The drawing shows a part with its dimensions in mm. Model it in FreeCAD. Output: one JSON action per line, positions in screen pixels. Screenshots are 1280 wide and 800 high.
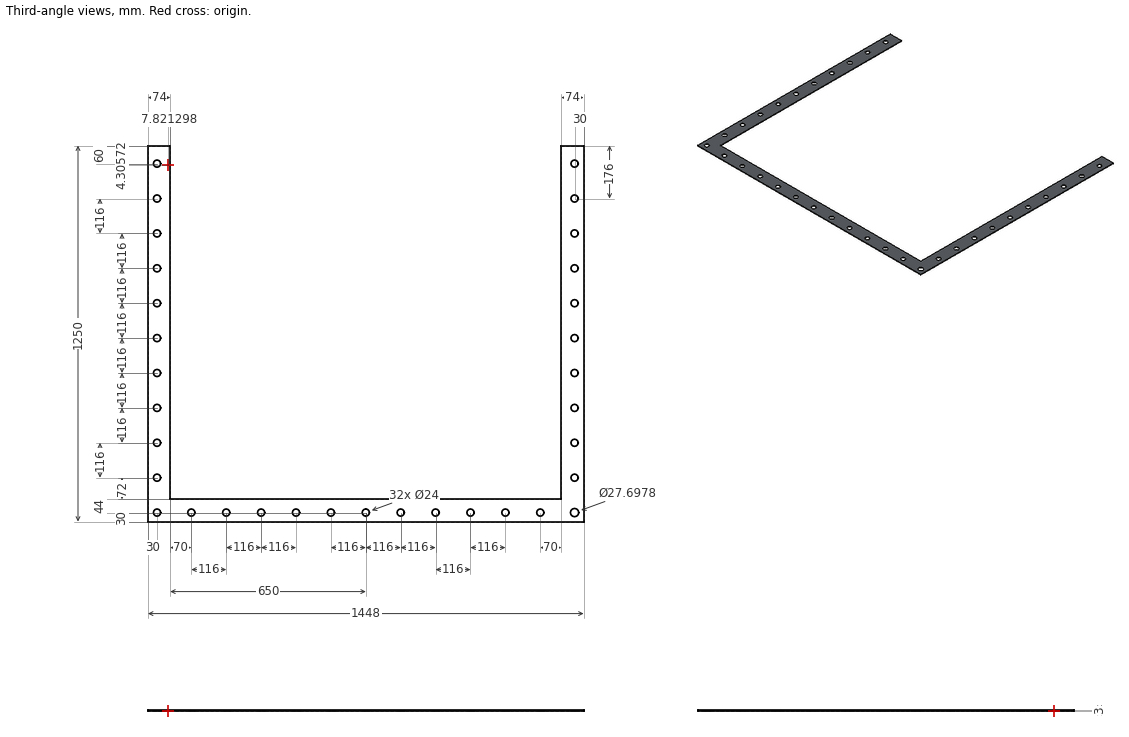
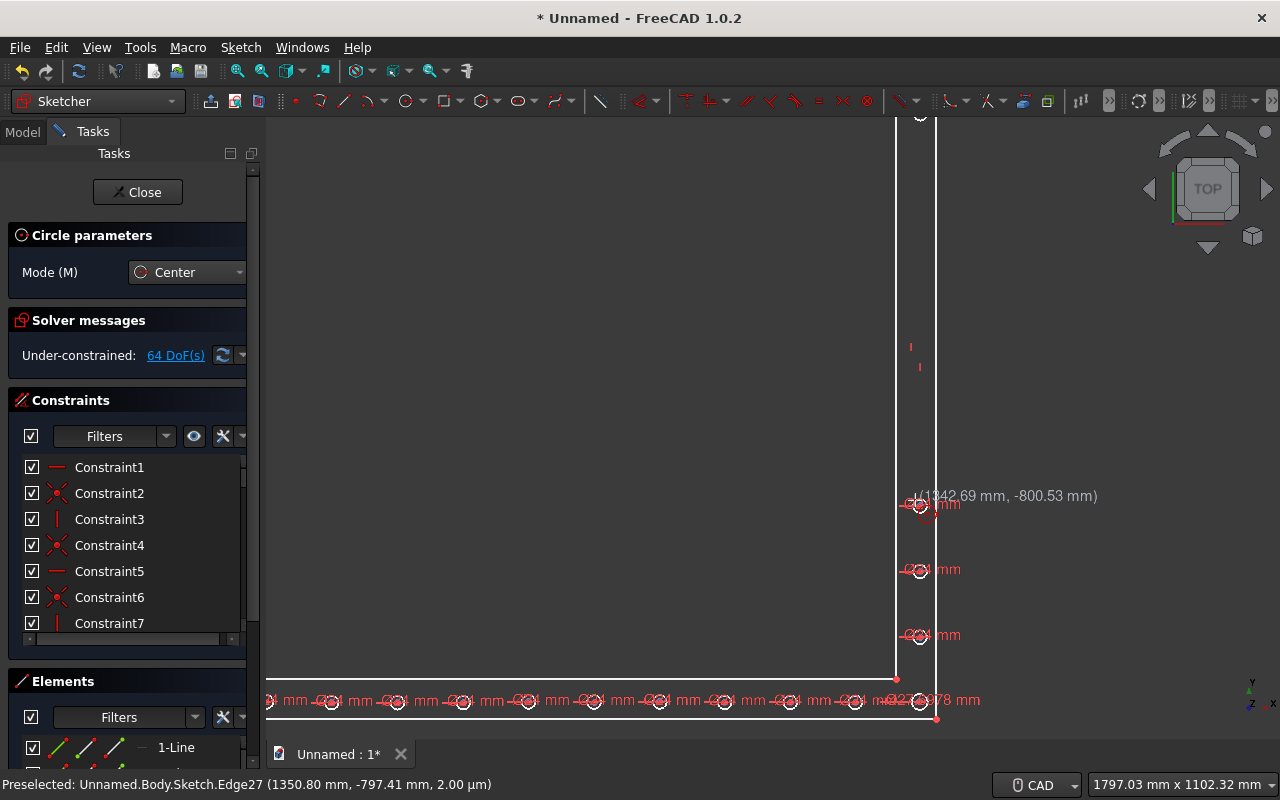
{"action": "scroll", "coordinate": [920, 440], "scroll_direction": "up", "scroll_amount": 7}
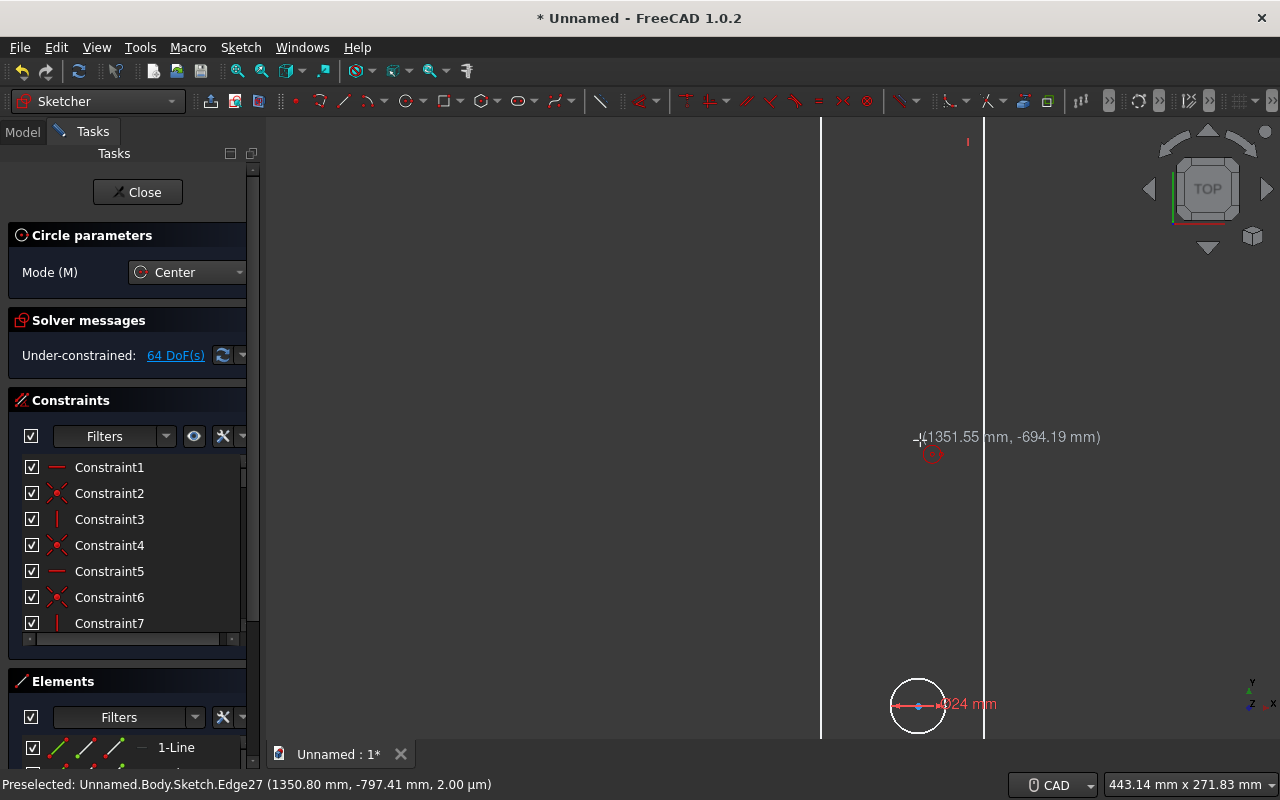
{"action": "scroll", "coordinate": [920, 474], "scroll_direction": "down", "scroll_amount": 10}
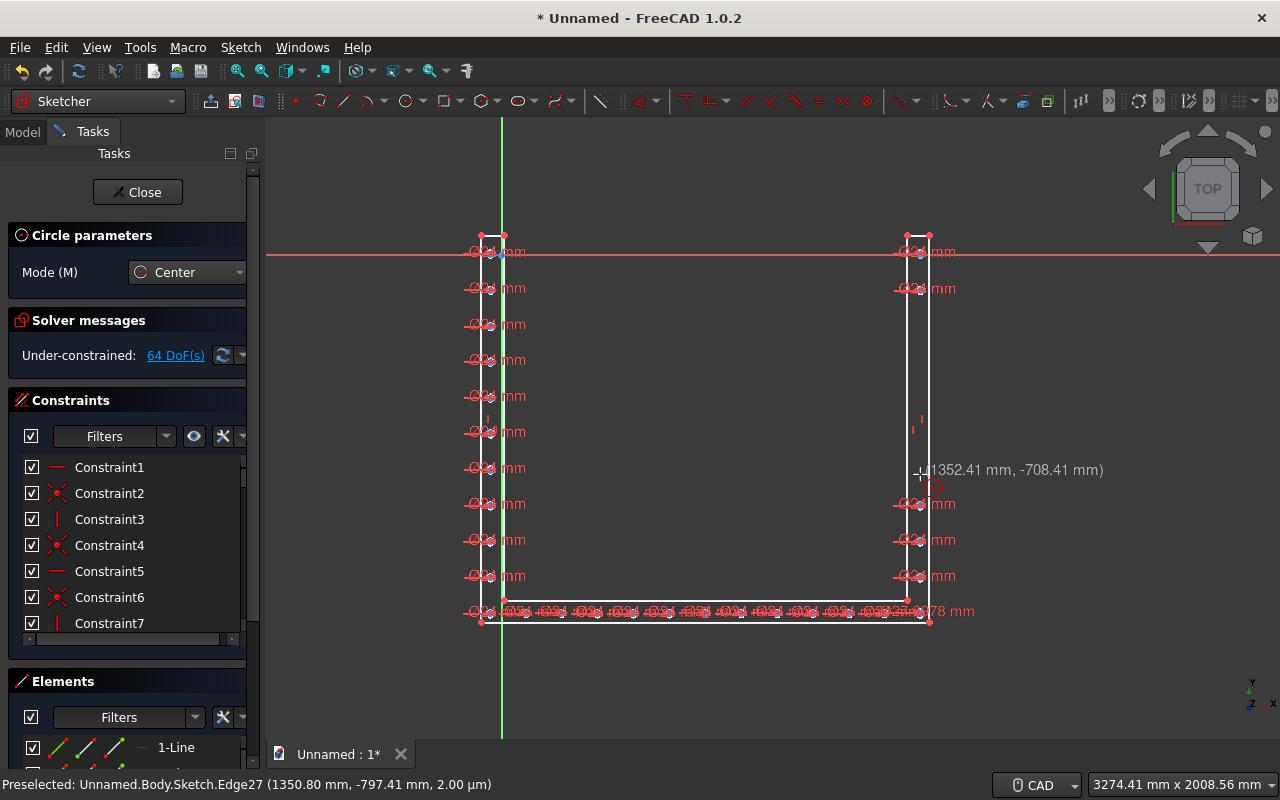
{"action": "scroll", "coordinate": [920, 469], "scroll_direction": "up", "scroll_amount": 3}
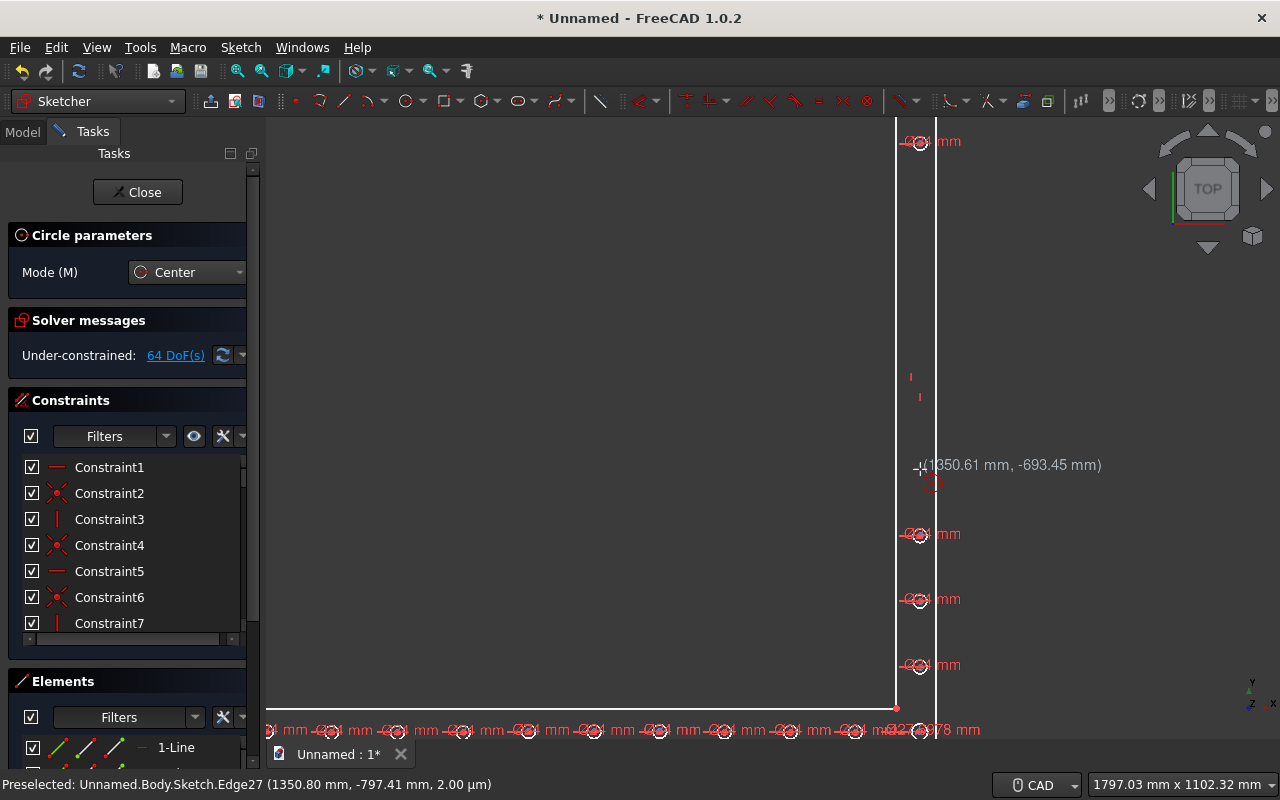
{"action": "left_click", "coordinate": [920, 469]}
{"action": "mouse_move", "coordinate": [915, 465]}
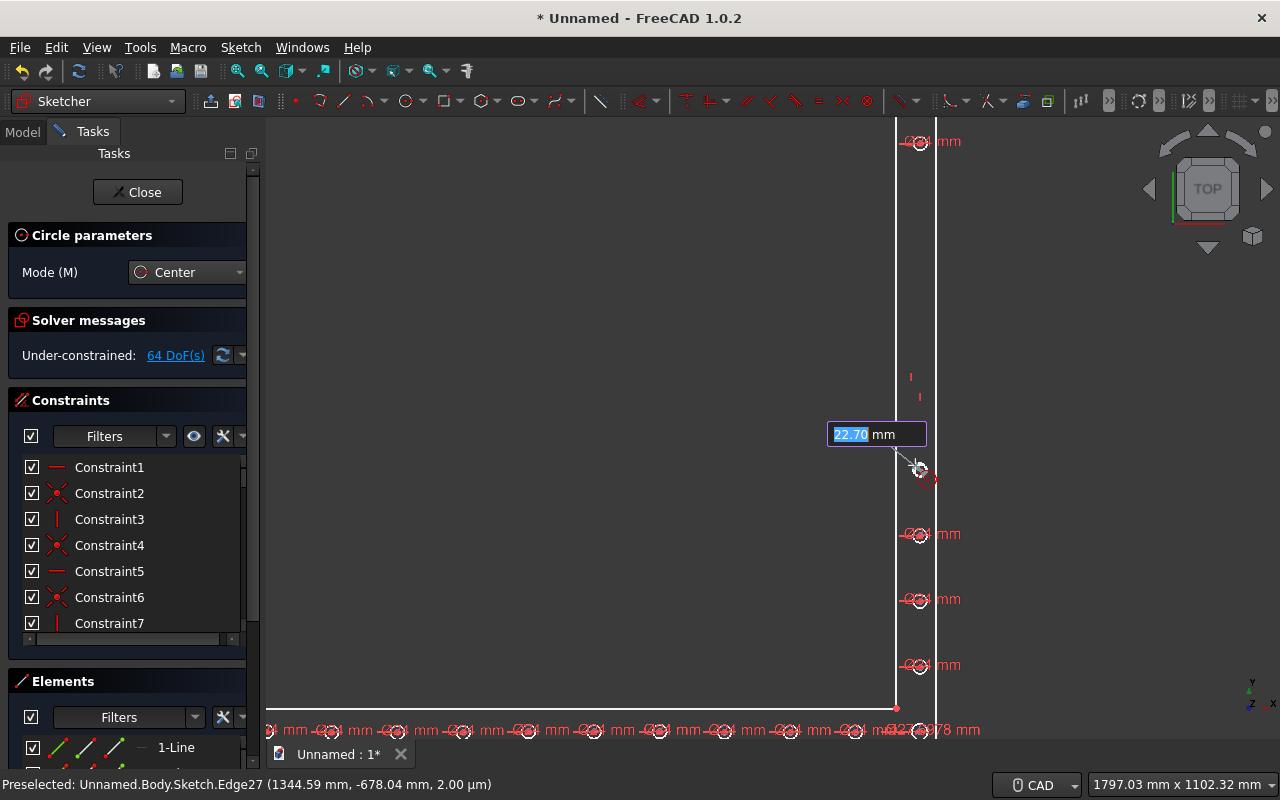
{"action": "type", "text": "24"}
{"action": "key", "text": "Return"}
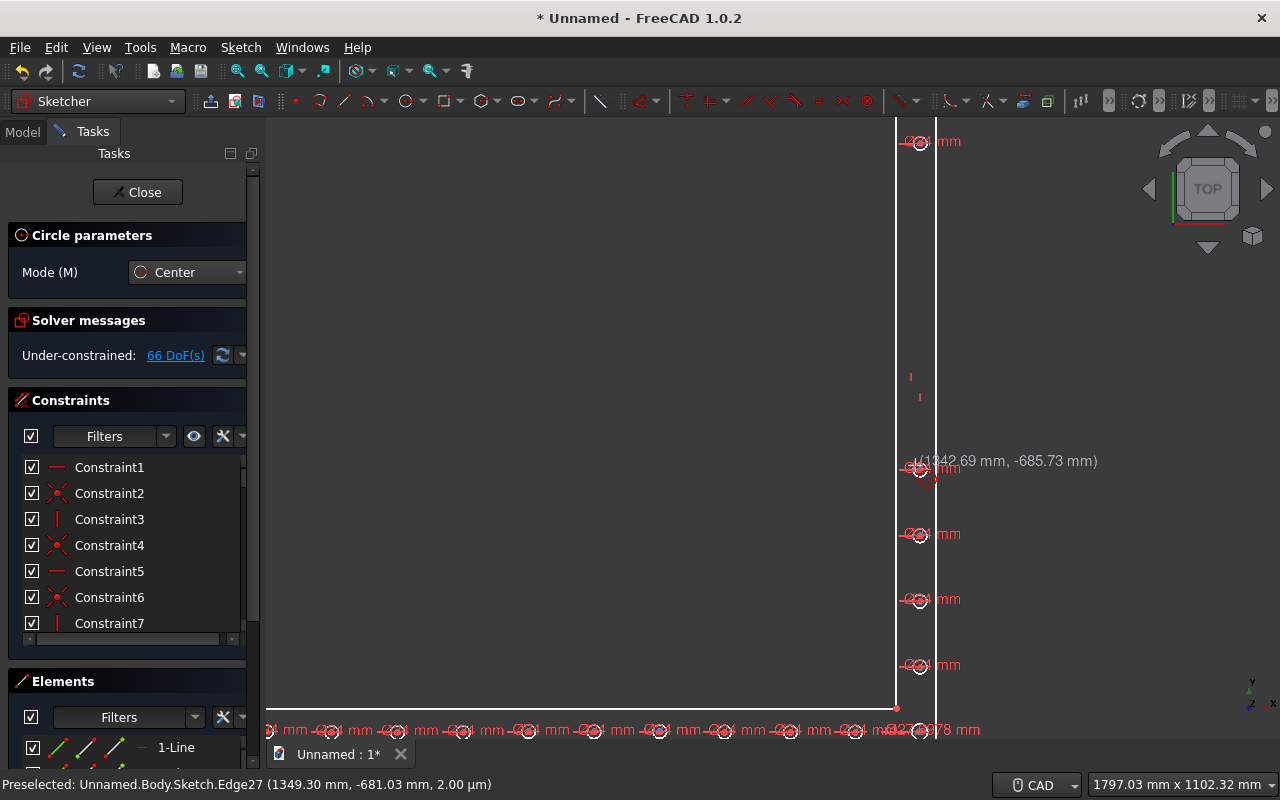
{"action": "scroll", "coordinate": [920, 404], "scroll_direction": "up", "scroll_amount": 7}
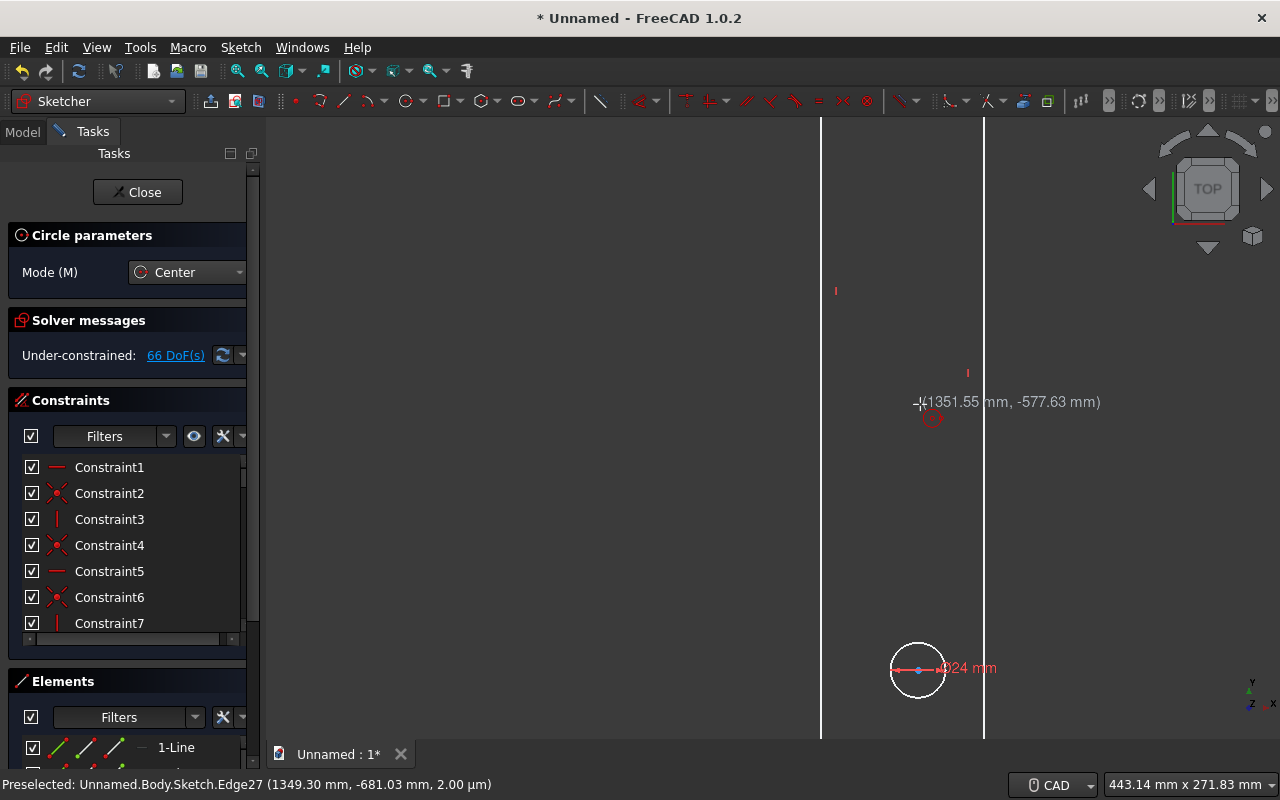
{"action": "scroll", "coordinate": [920, 437], "scroll_direction": "down", "scroll_amount": 10}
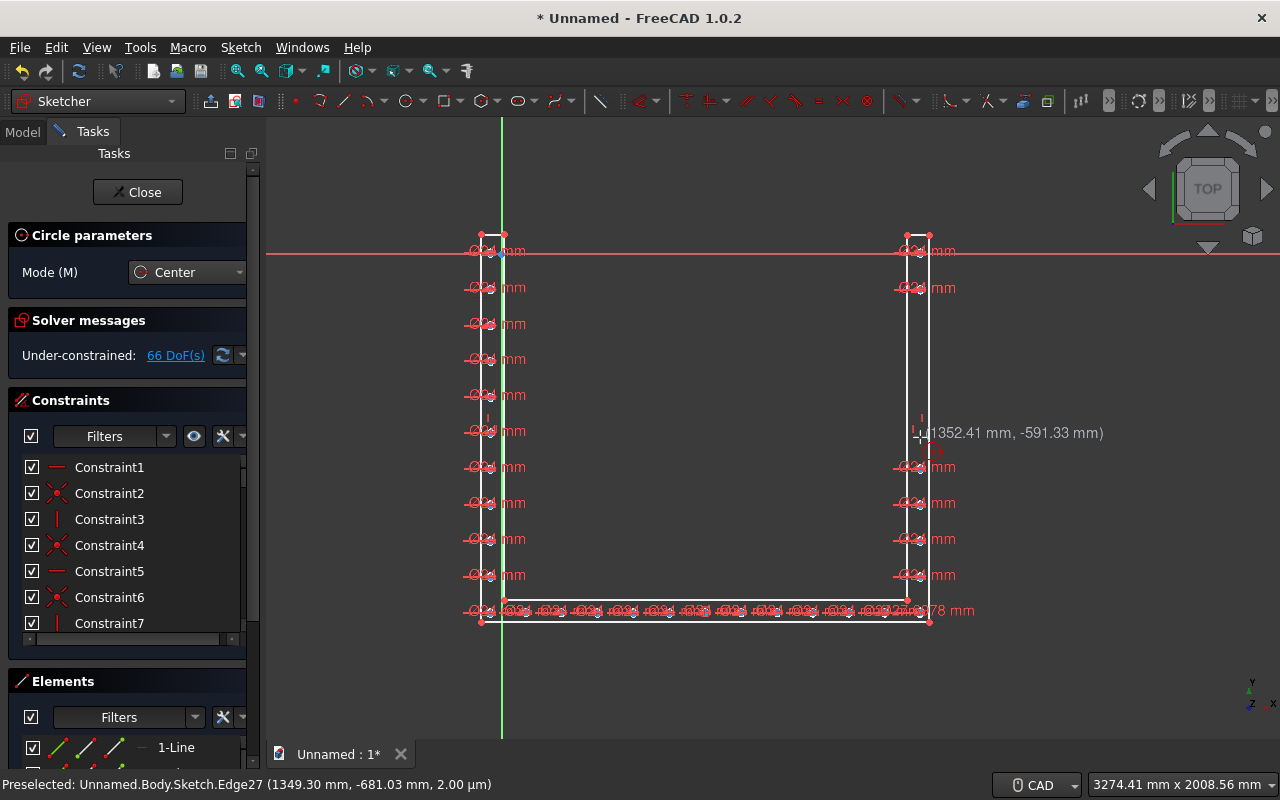
{"action": "scroll", "coordinate": [920, 433], "scroll_direction": "up", "scroll_amount": 3}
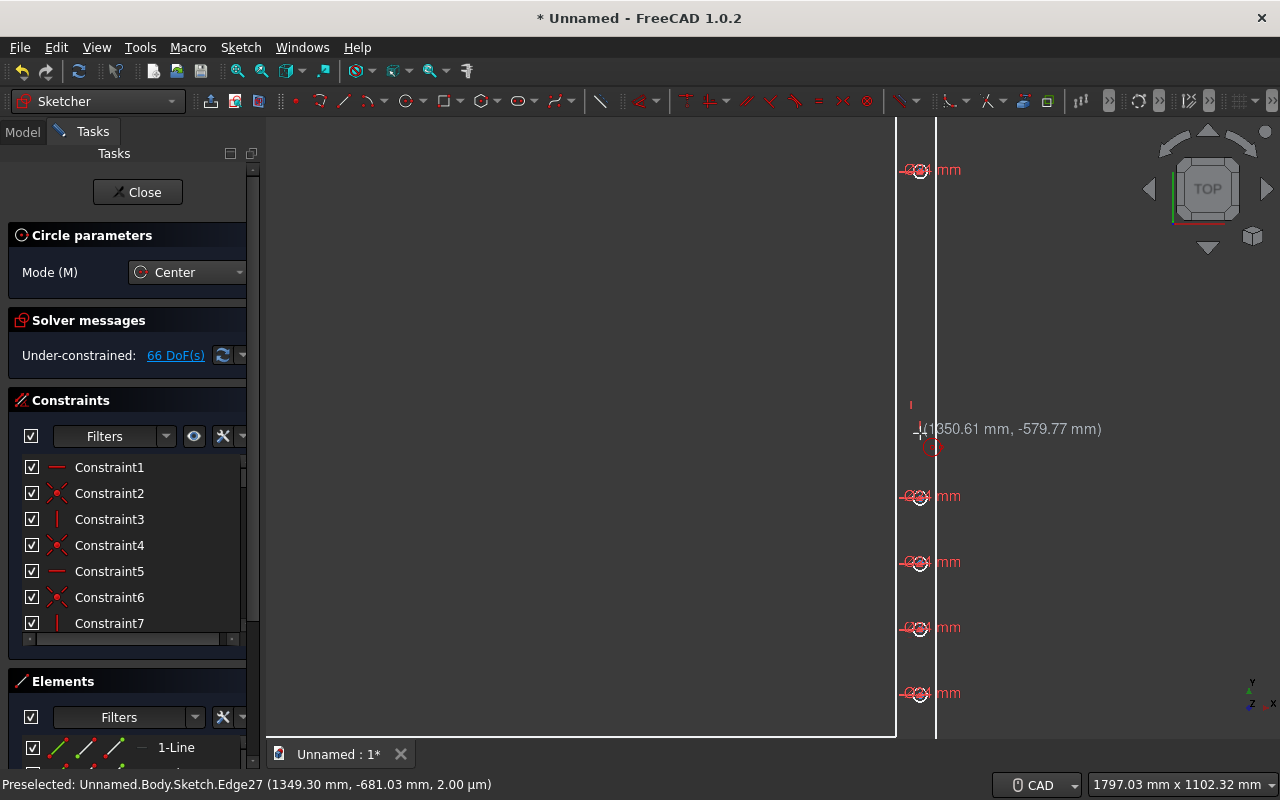
{"action": "left_click", "coordinate": [920, 432]}
{"action": "mouse_move", "coordinate": [915, 427]}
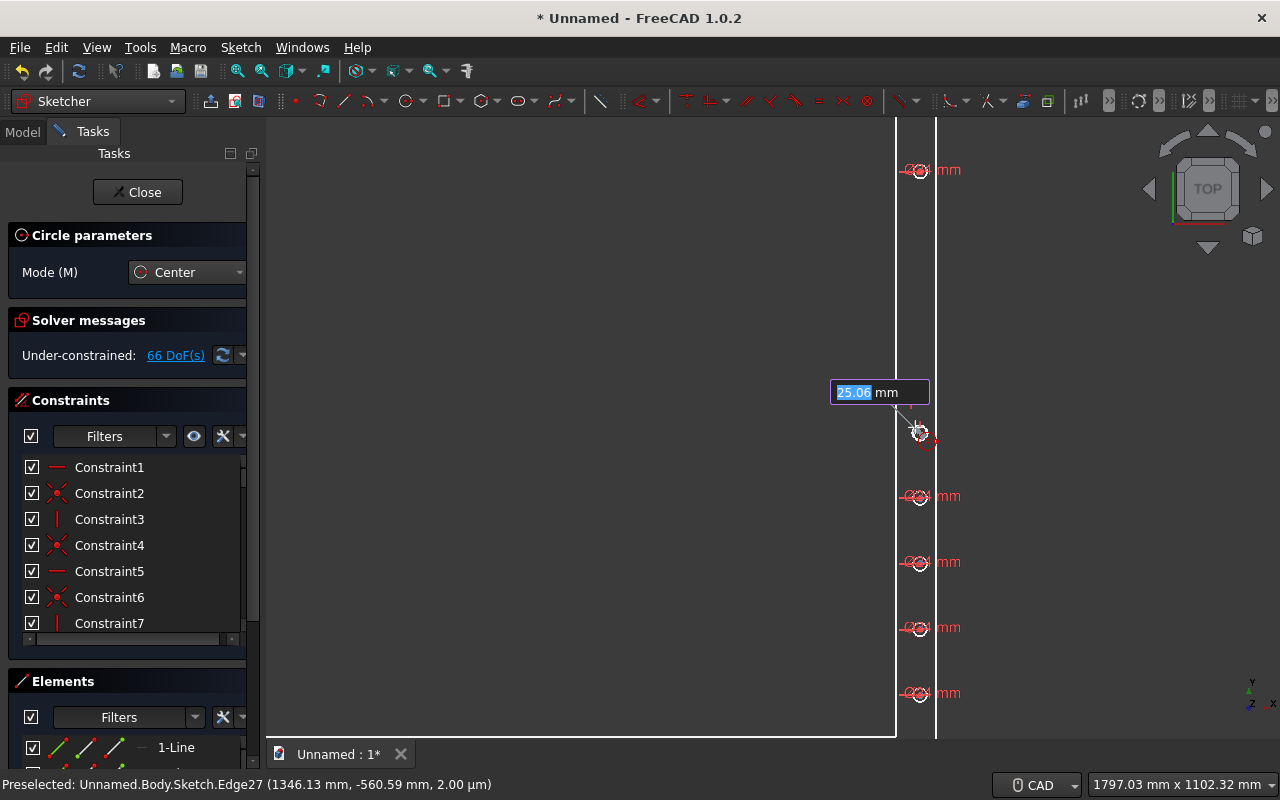
{"action": "type", "text": "24"}
{"action": "key", "text": "Return"}